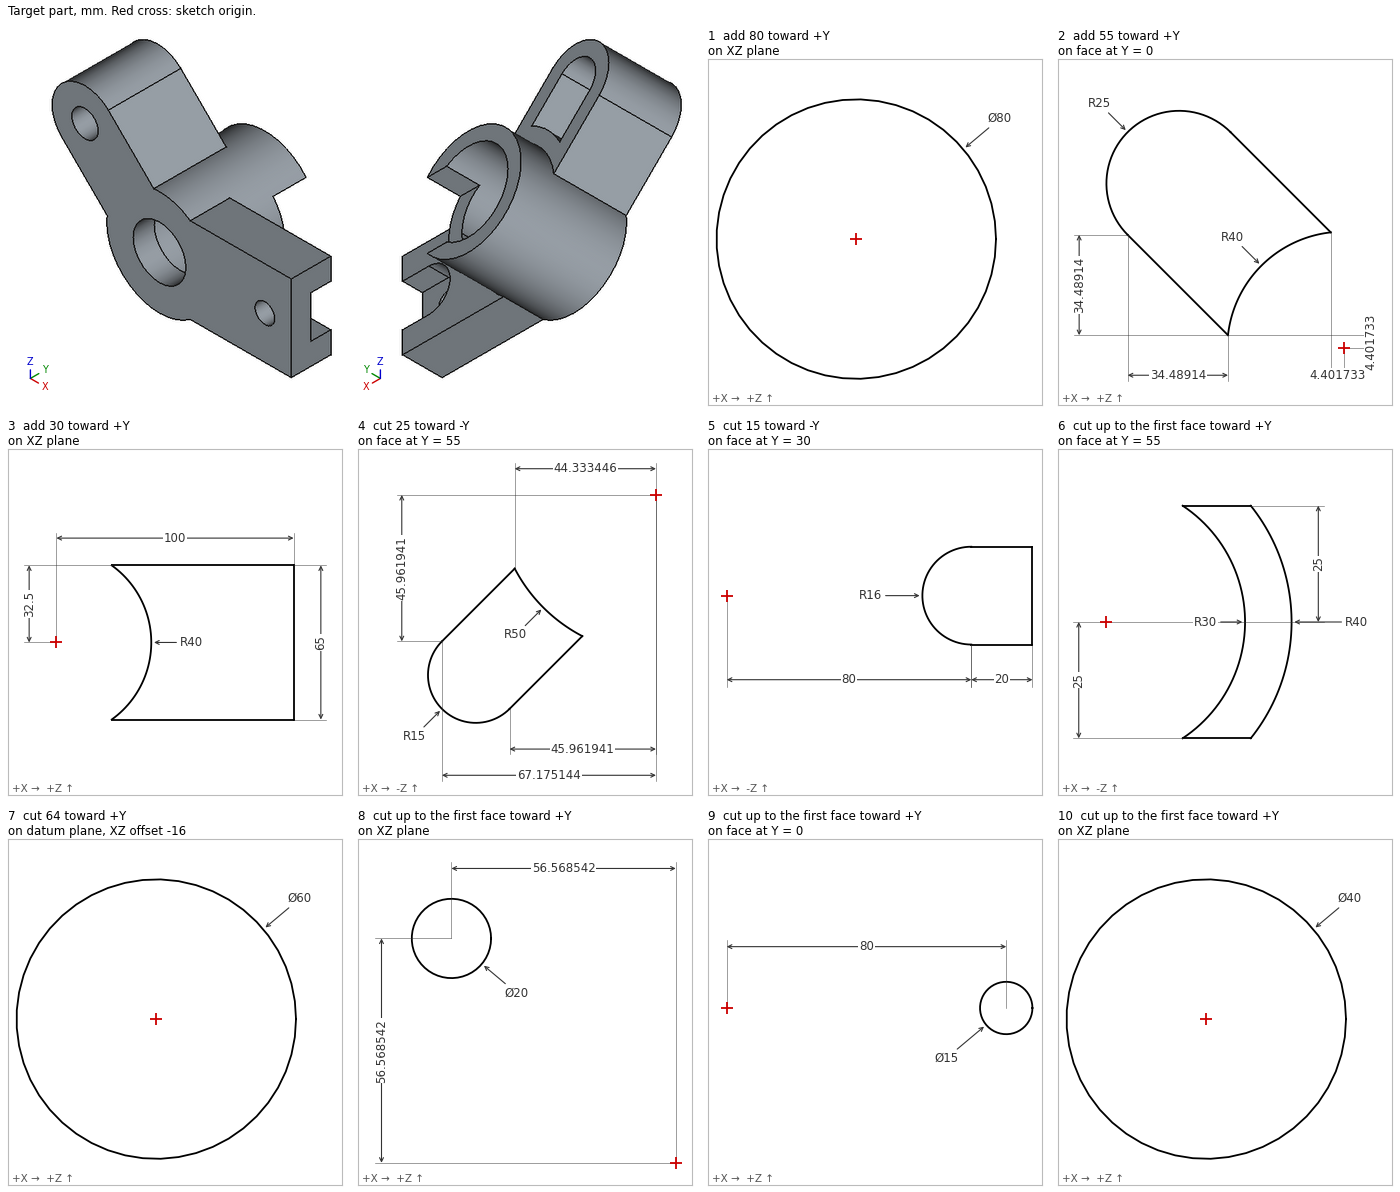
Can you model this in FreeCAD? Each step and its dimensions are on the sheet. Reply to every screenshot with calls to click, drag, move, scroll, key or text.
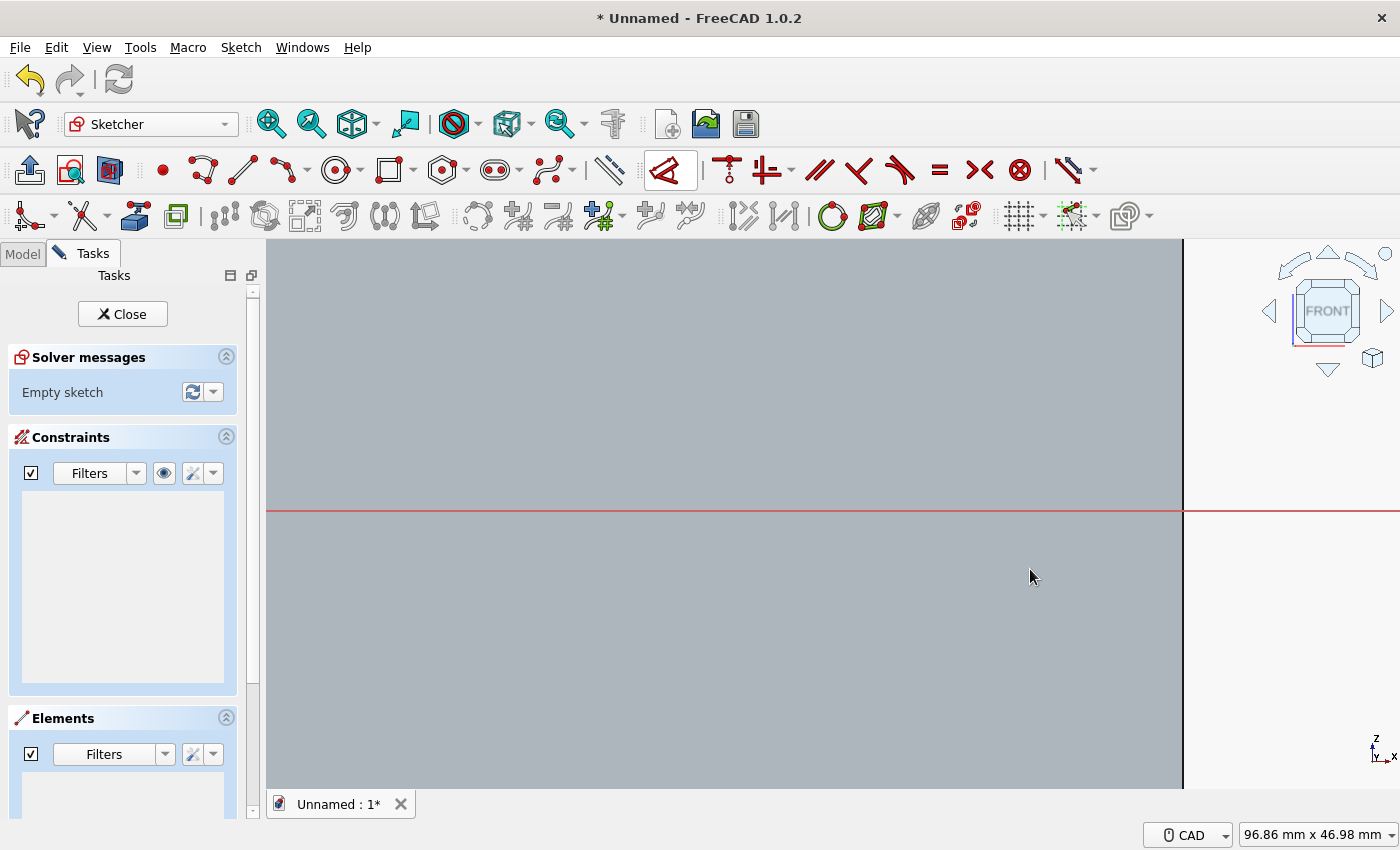
click(336, 170)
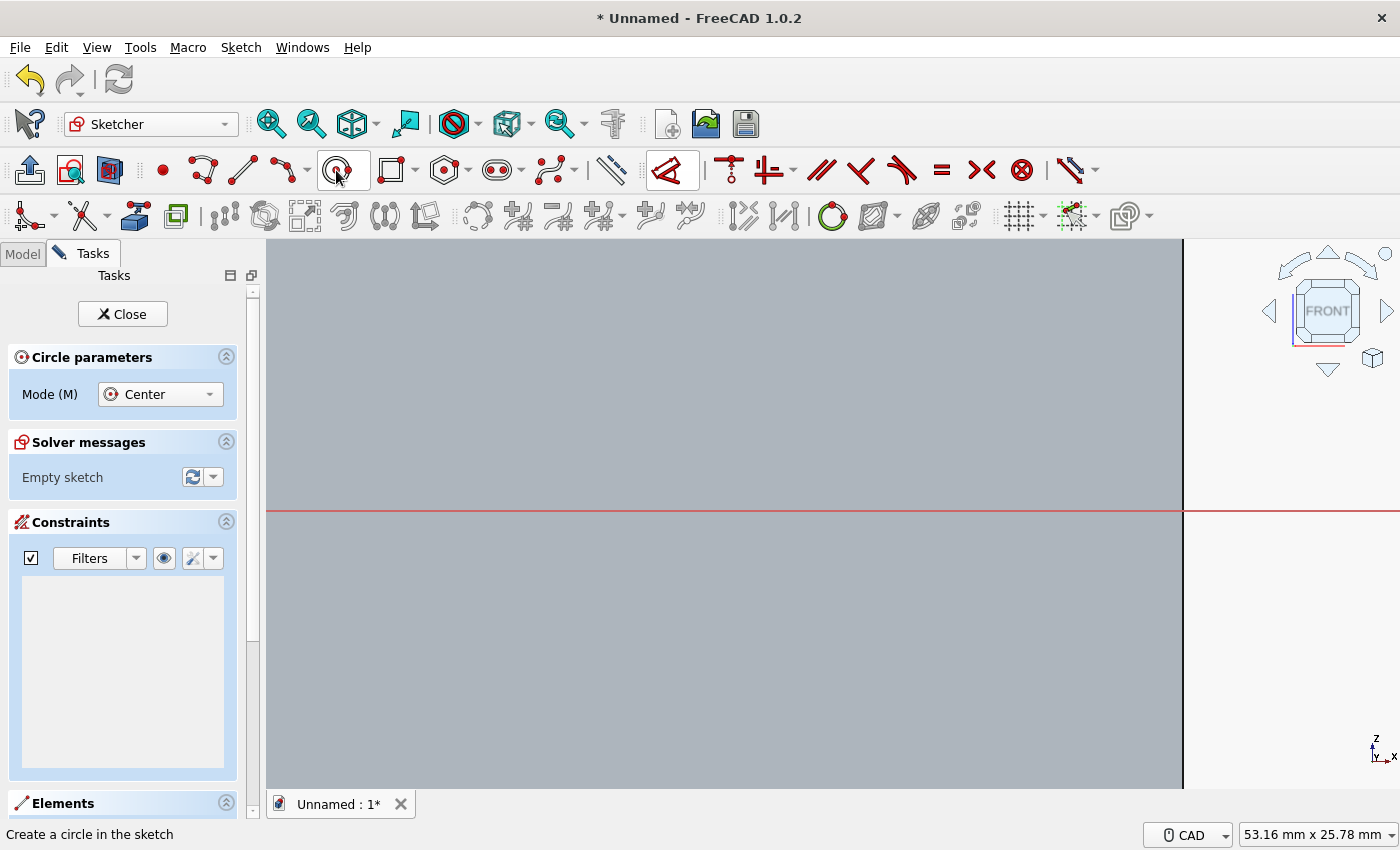
click(757, 511)
click(870, 398)
key(Escape)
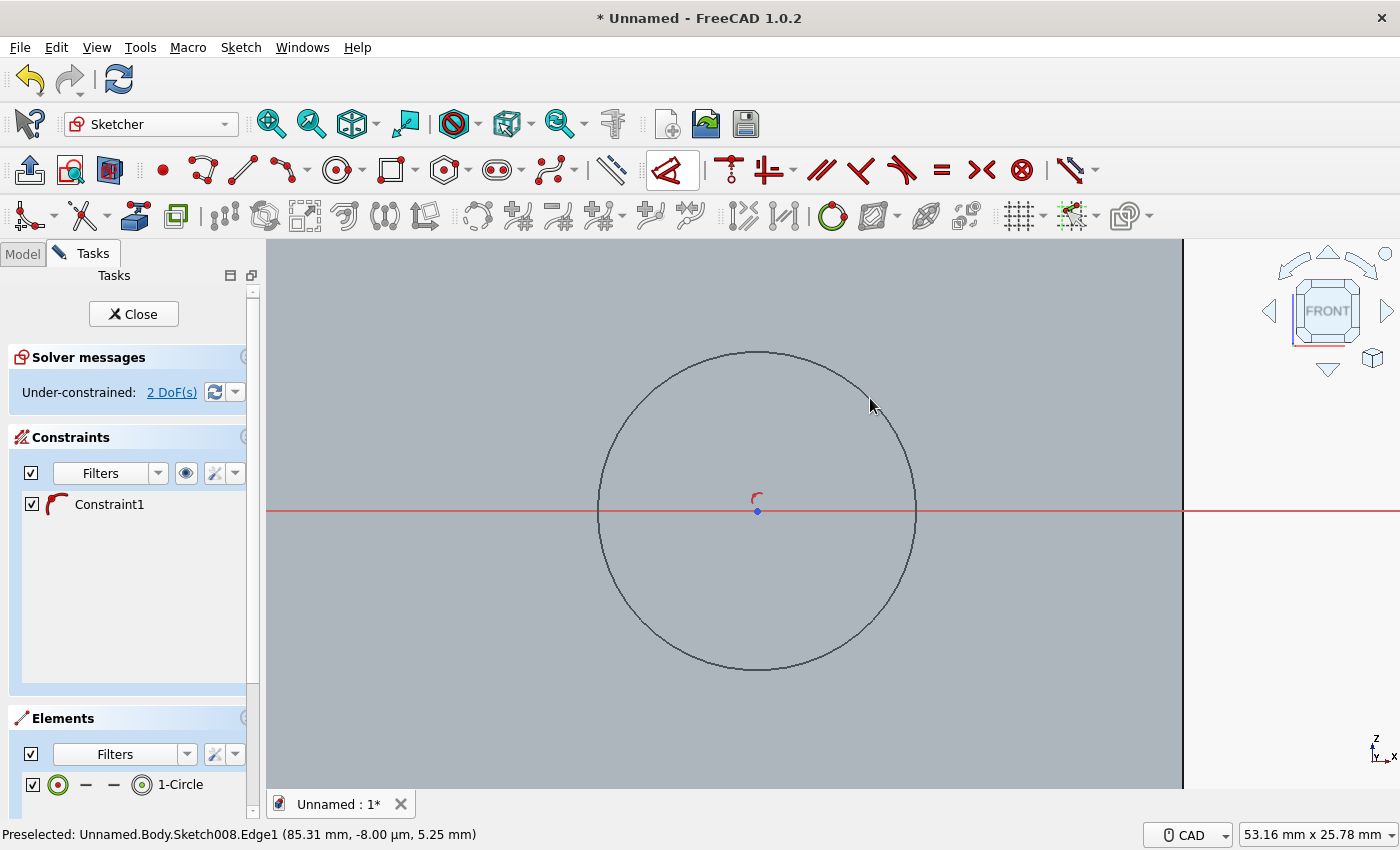
click(869, 398)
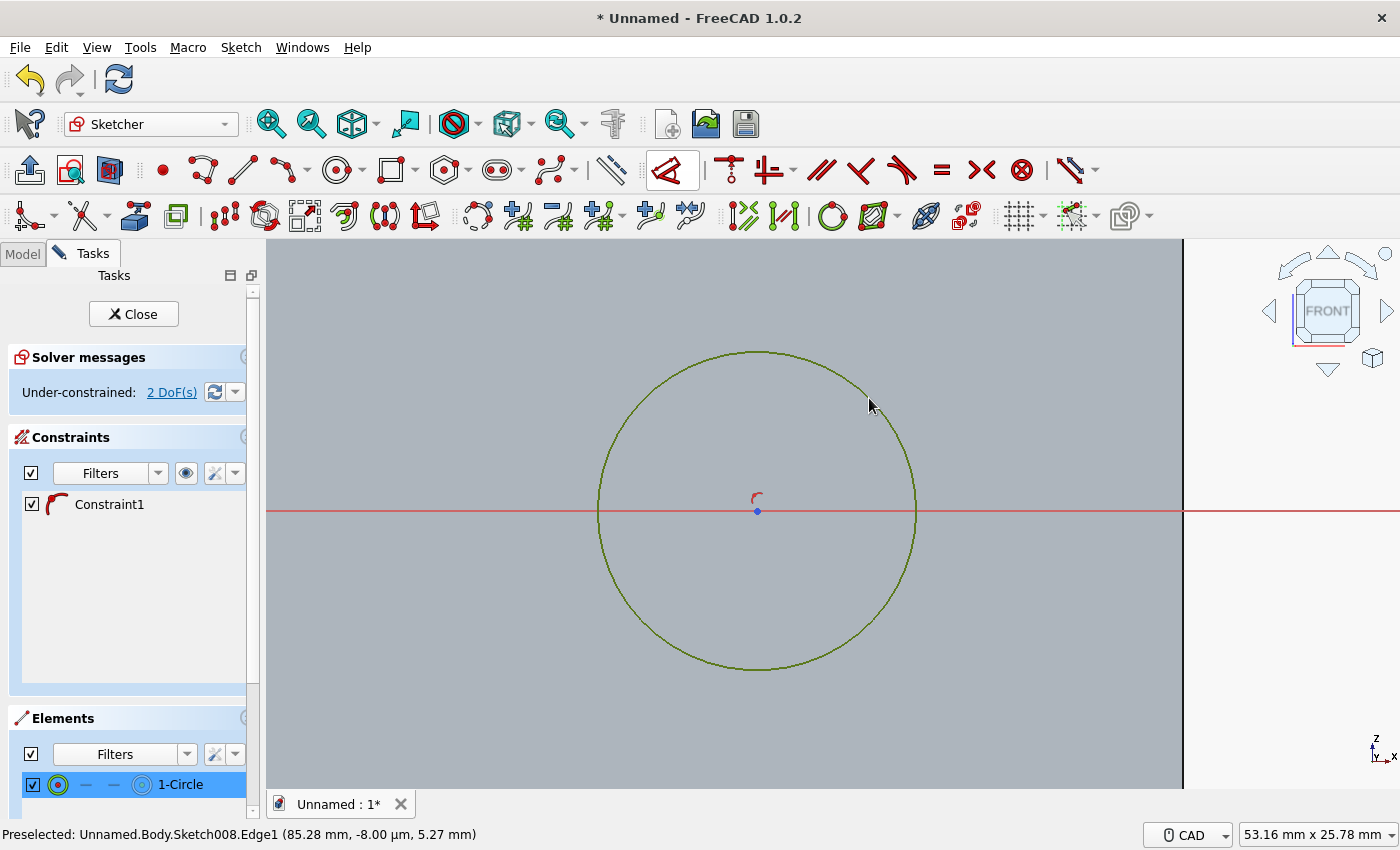
click(694, 170)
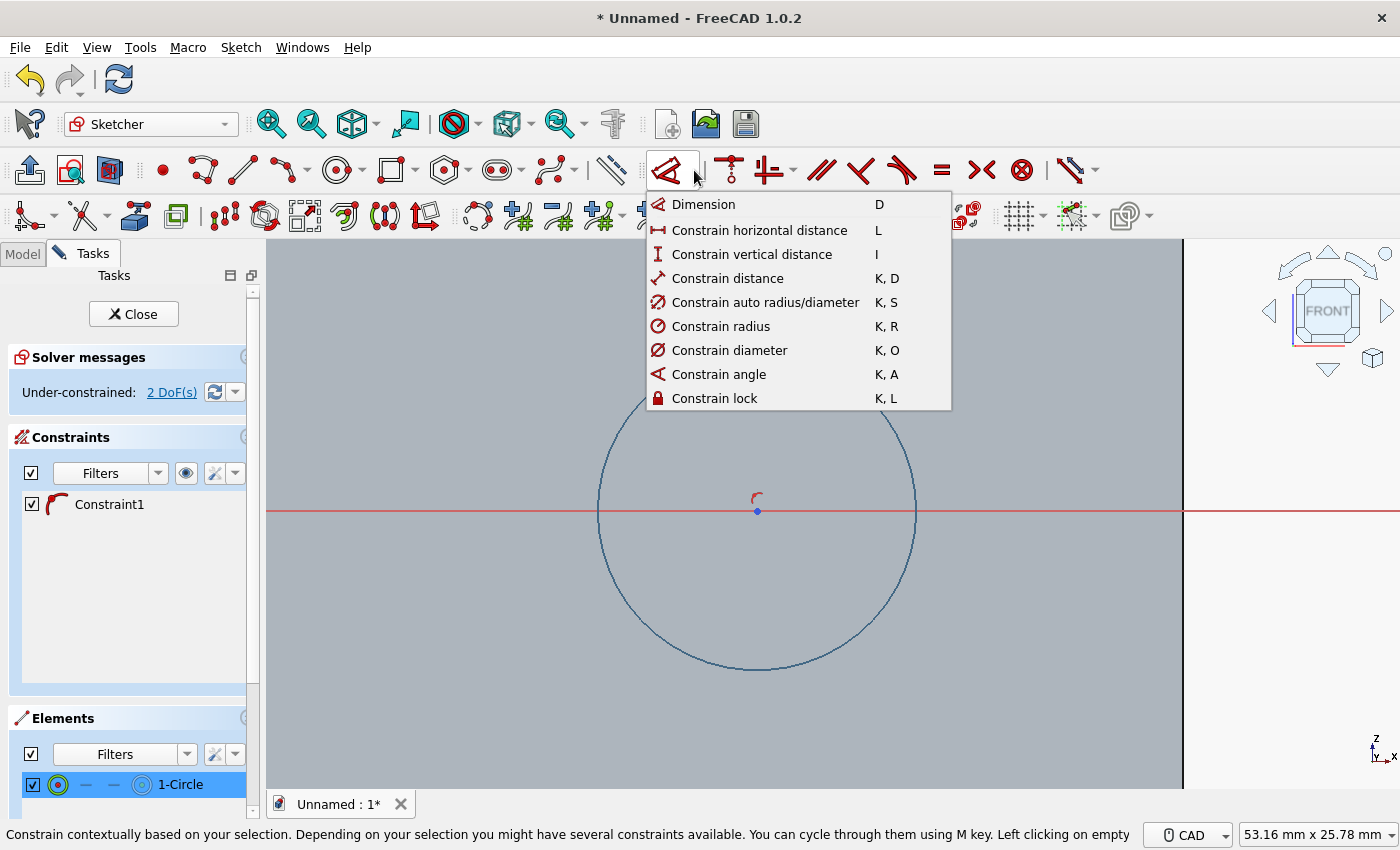
click(799, 350)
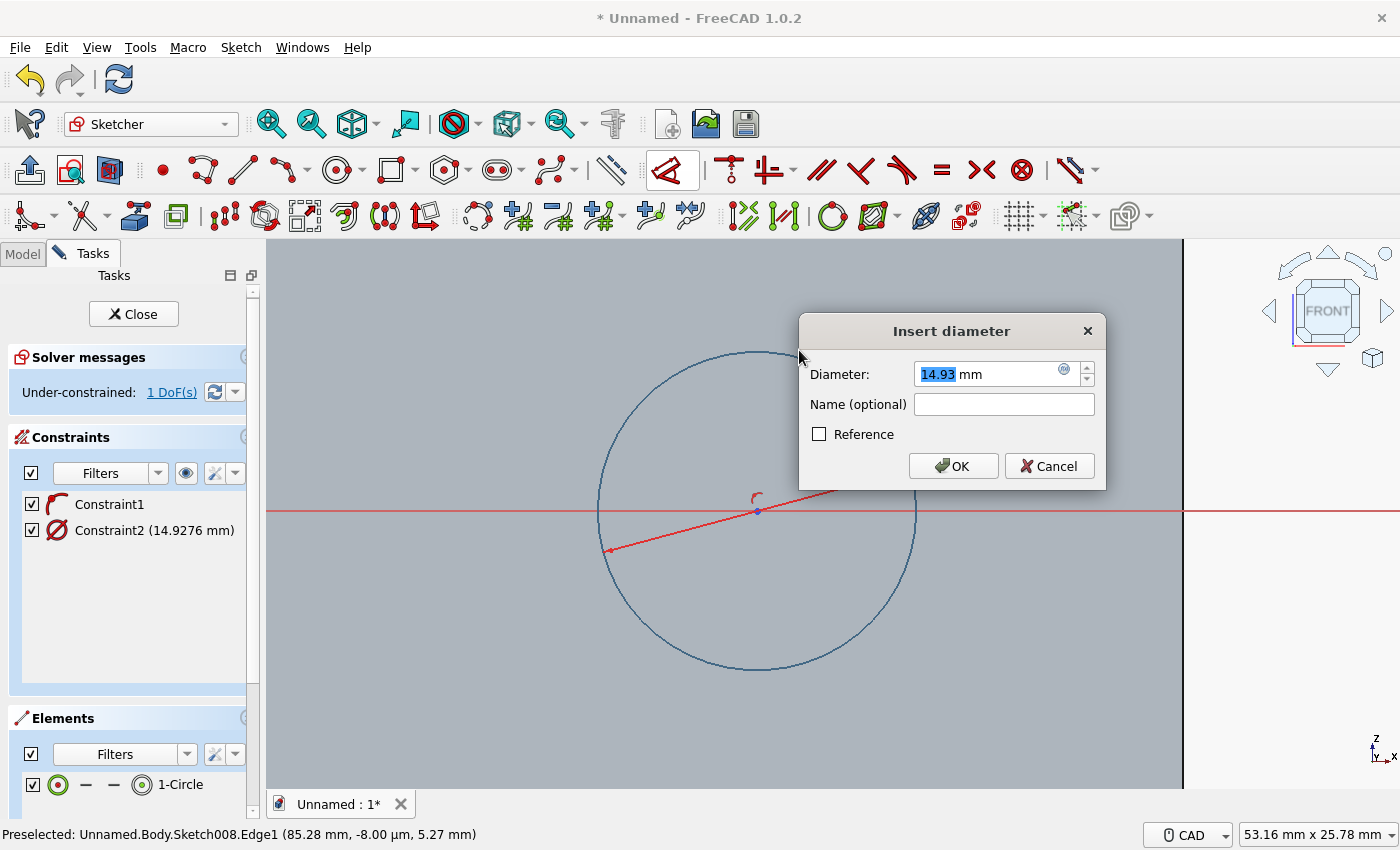
text(15)
key(Return)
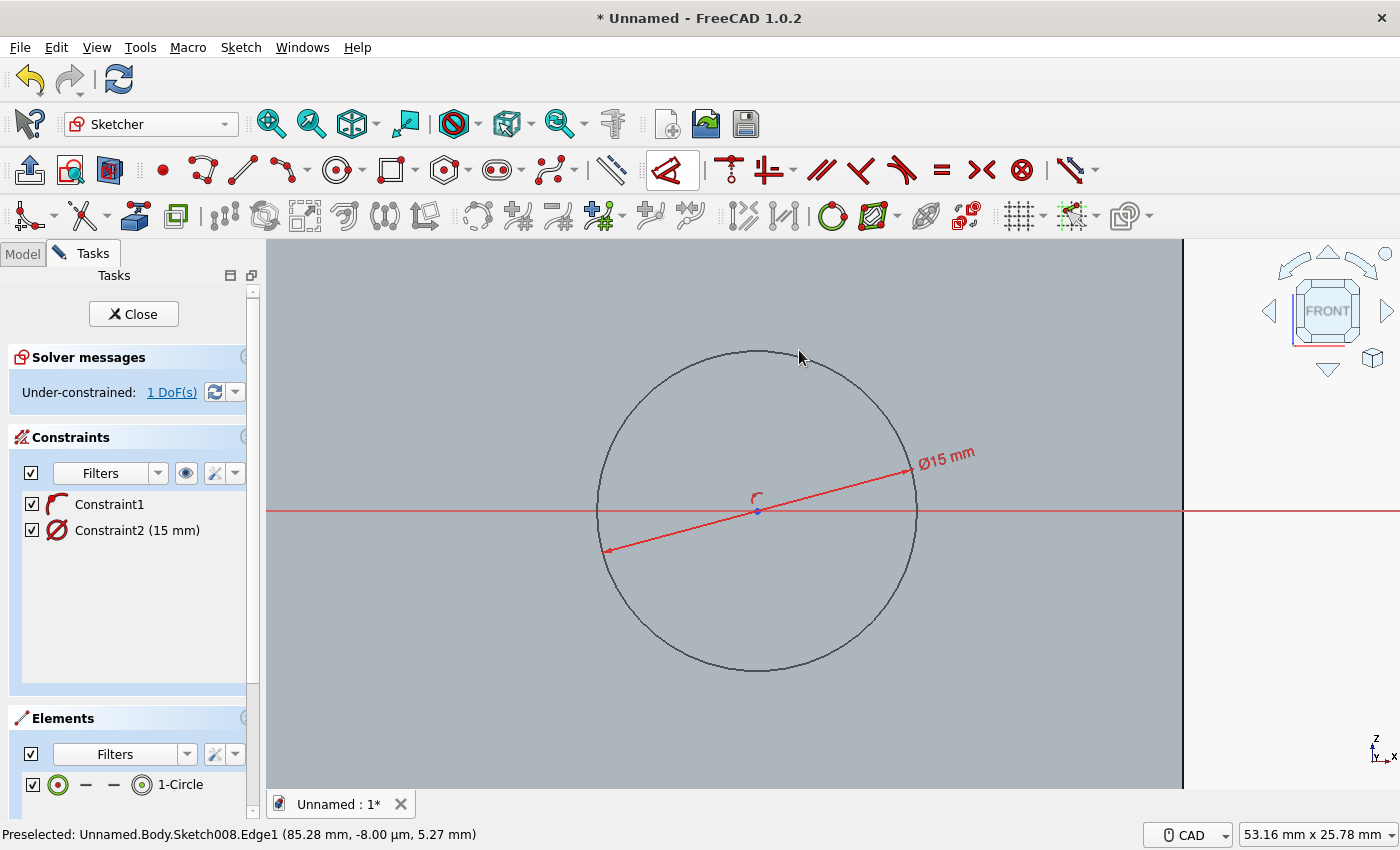
click(757, 511)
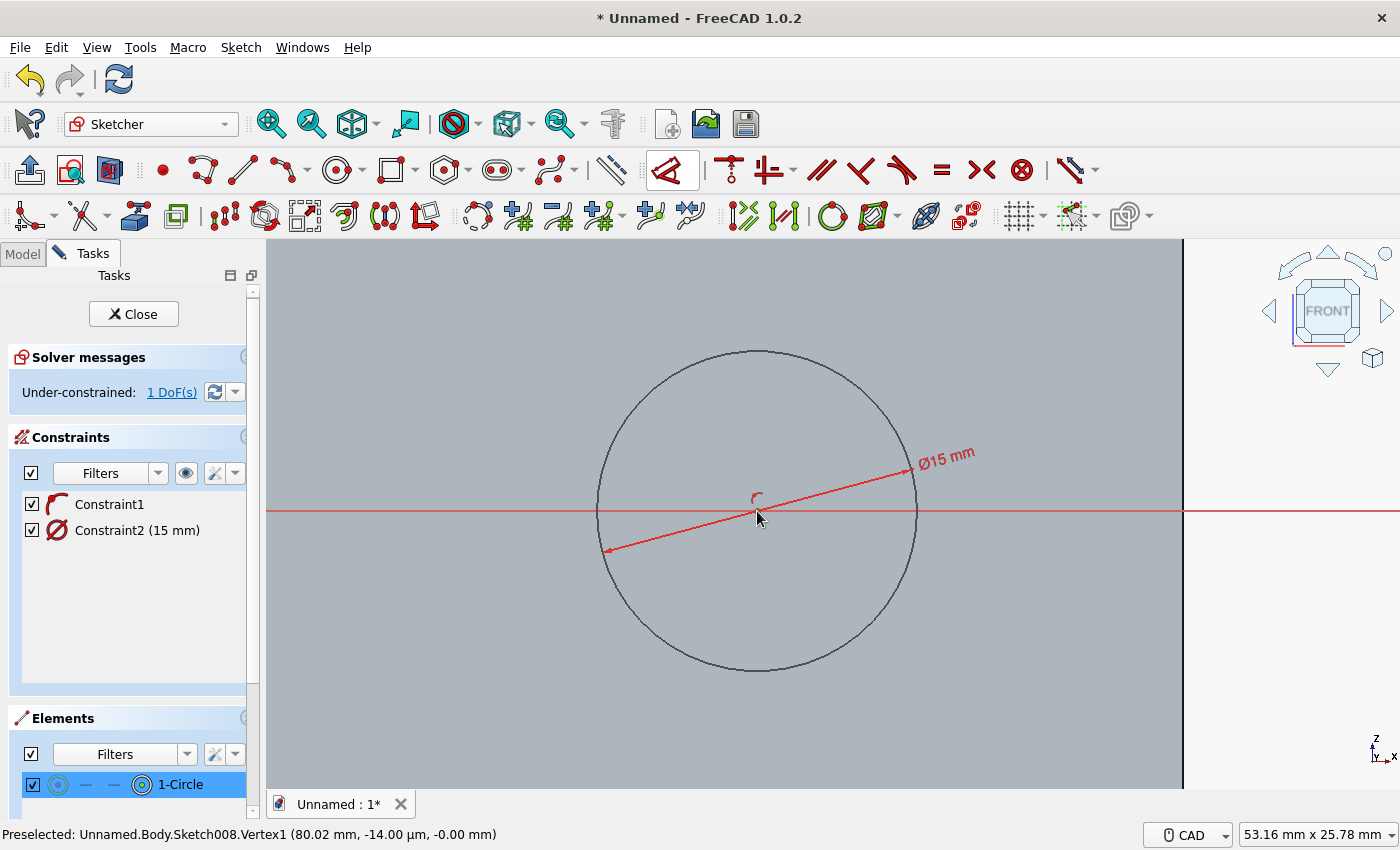
click(694, 170)